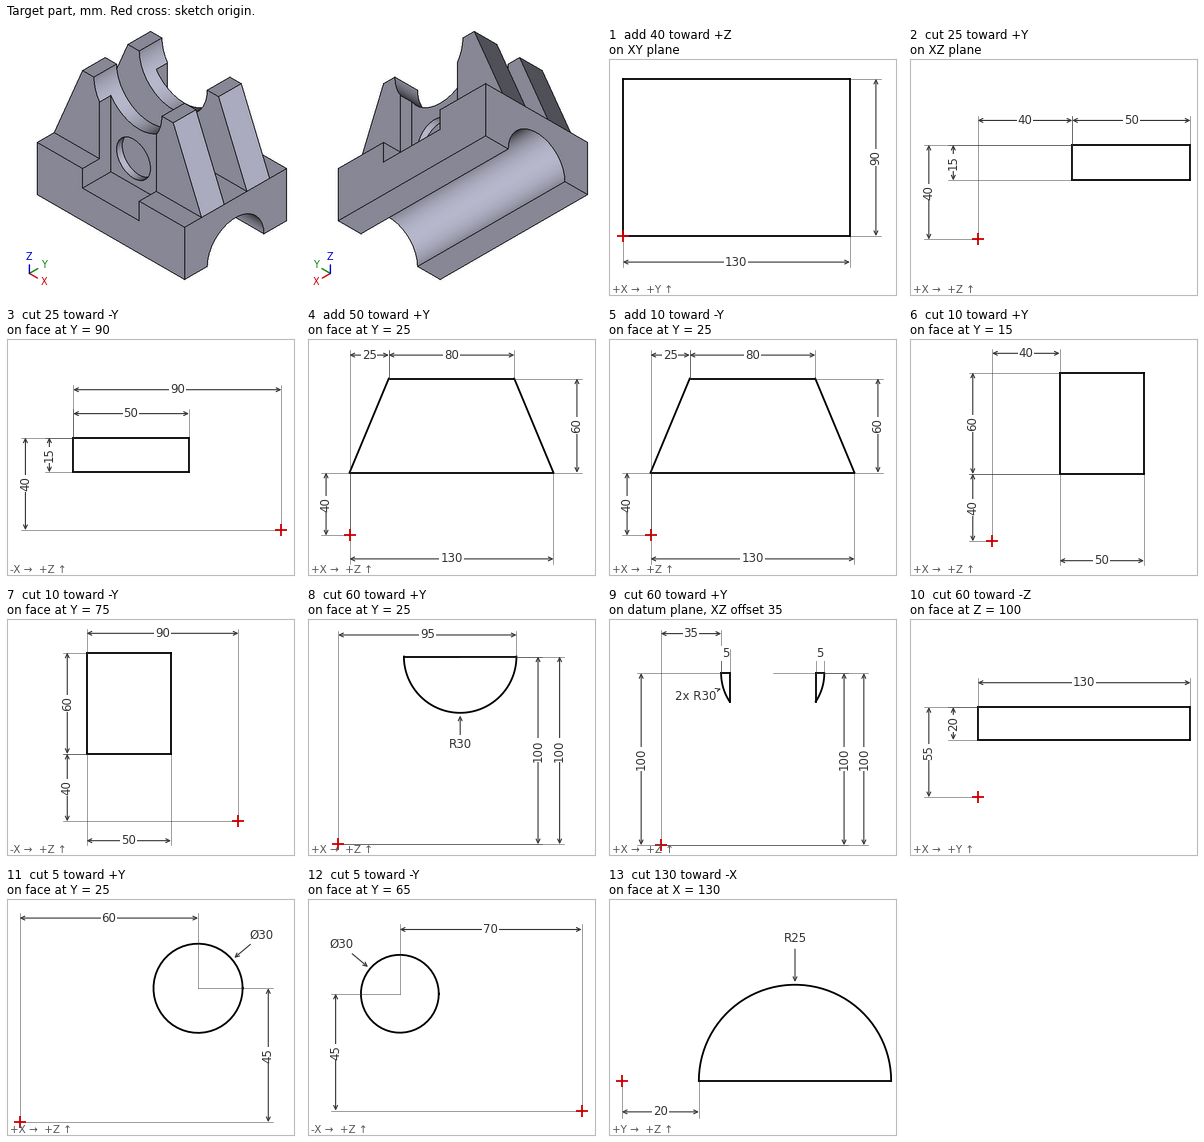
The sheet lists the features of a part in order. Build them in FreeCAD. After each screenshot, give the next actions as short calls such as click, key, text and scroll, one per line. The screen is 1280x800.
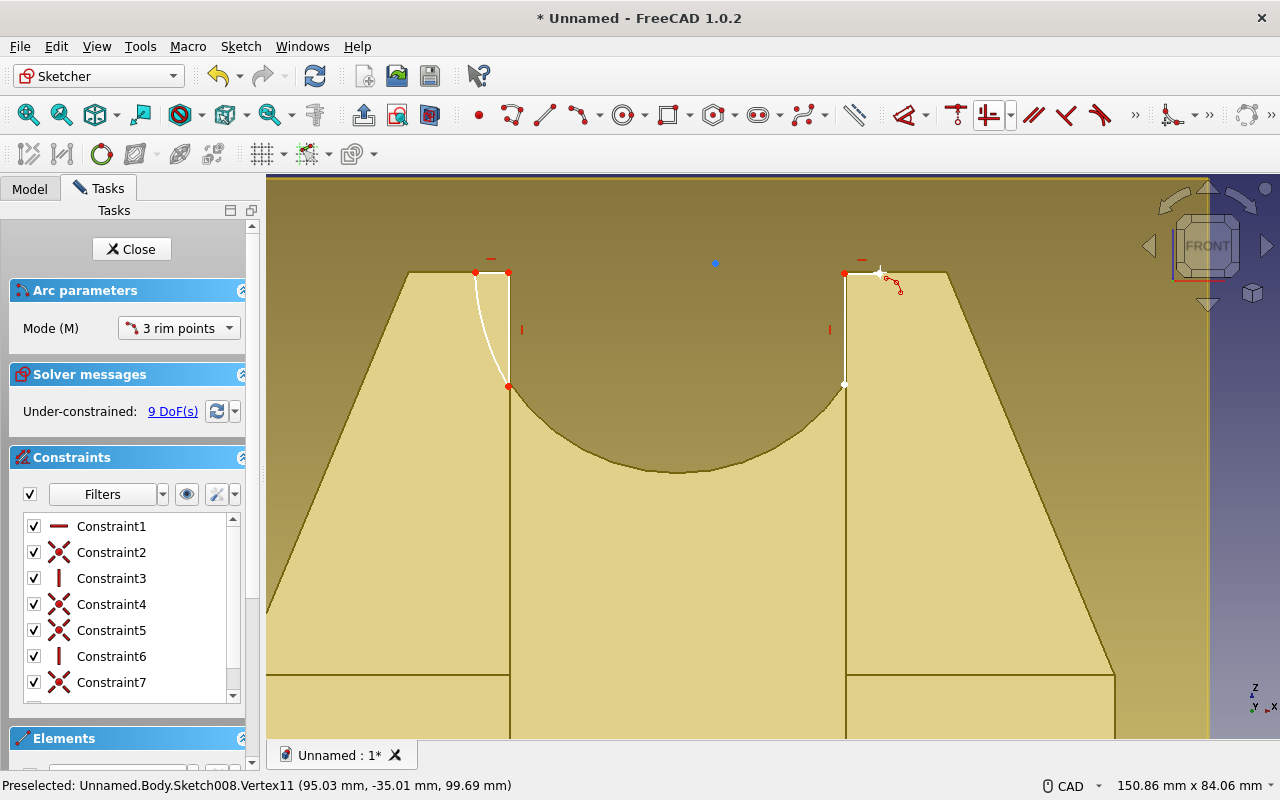
click(880, 274)
click(845, 385)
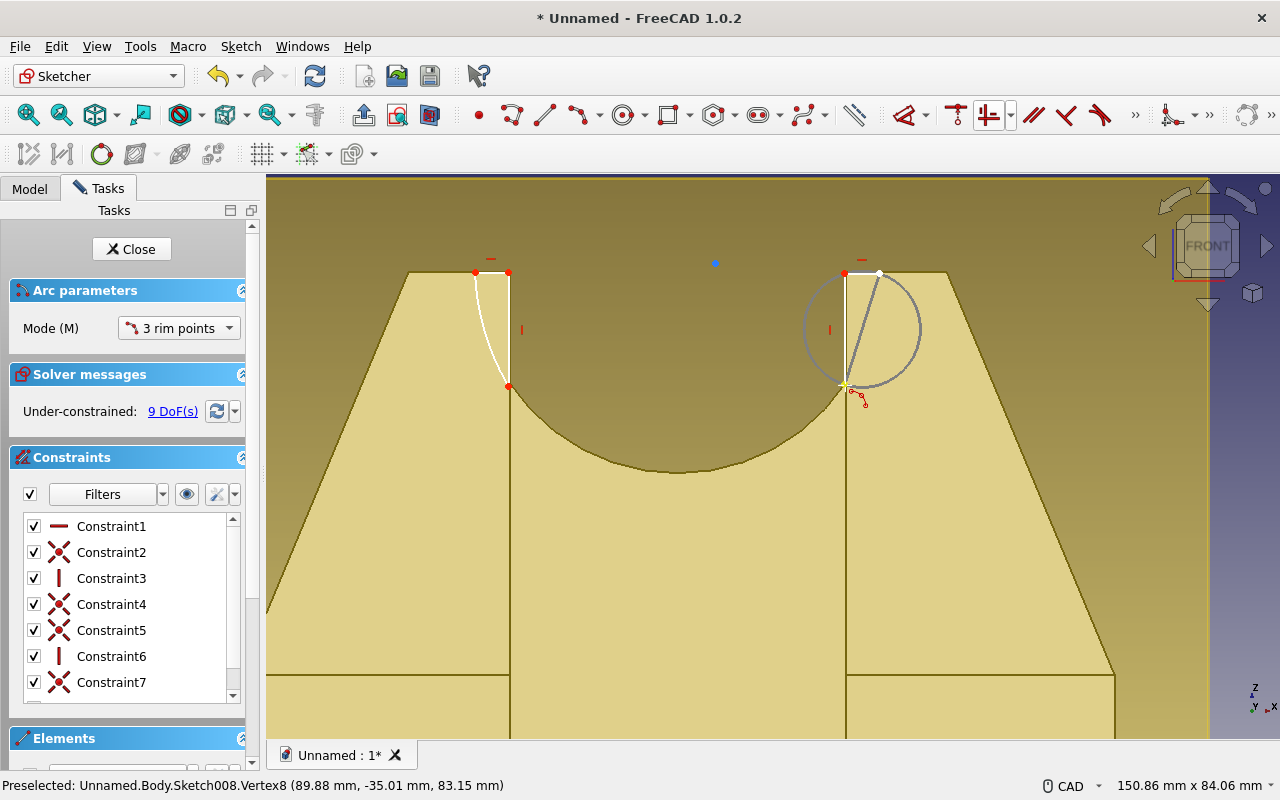
scroll(871, 330, up, 4)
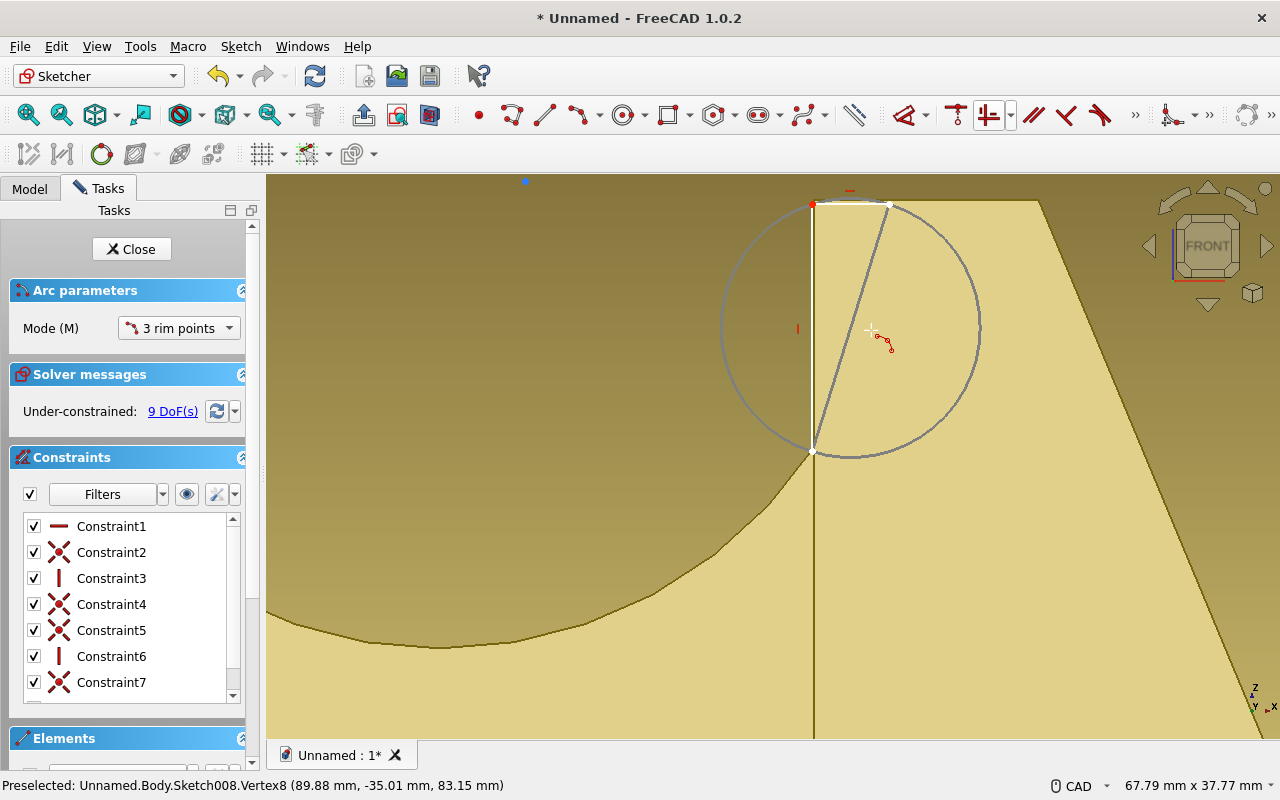
click(870, 329)
key(Escape)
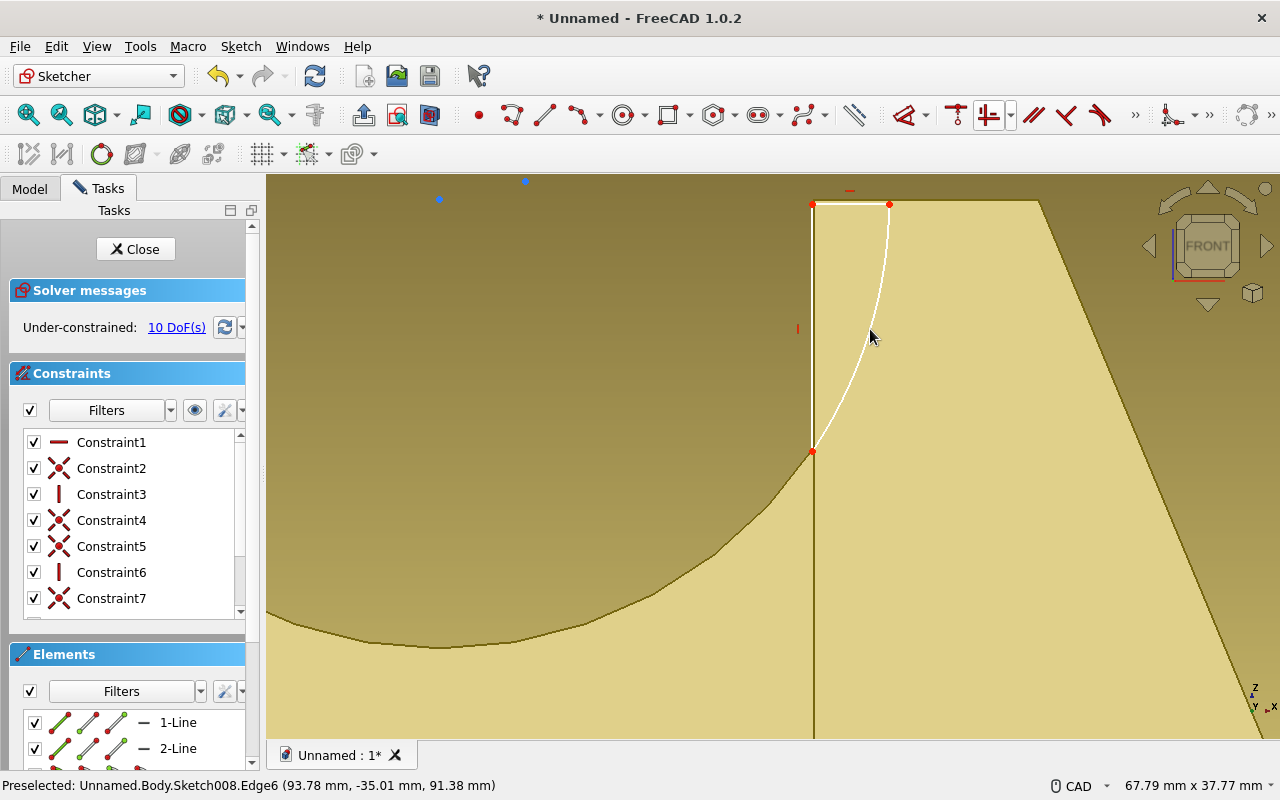
scroll(877, 296, down, 7)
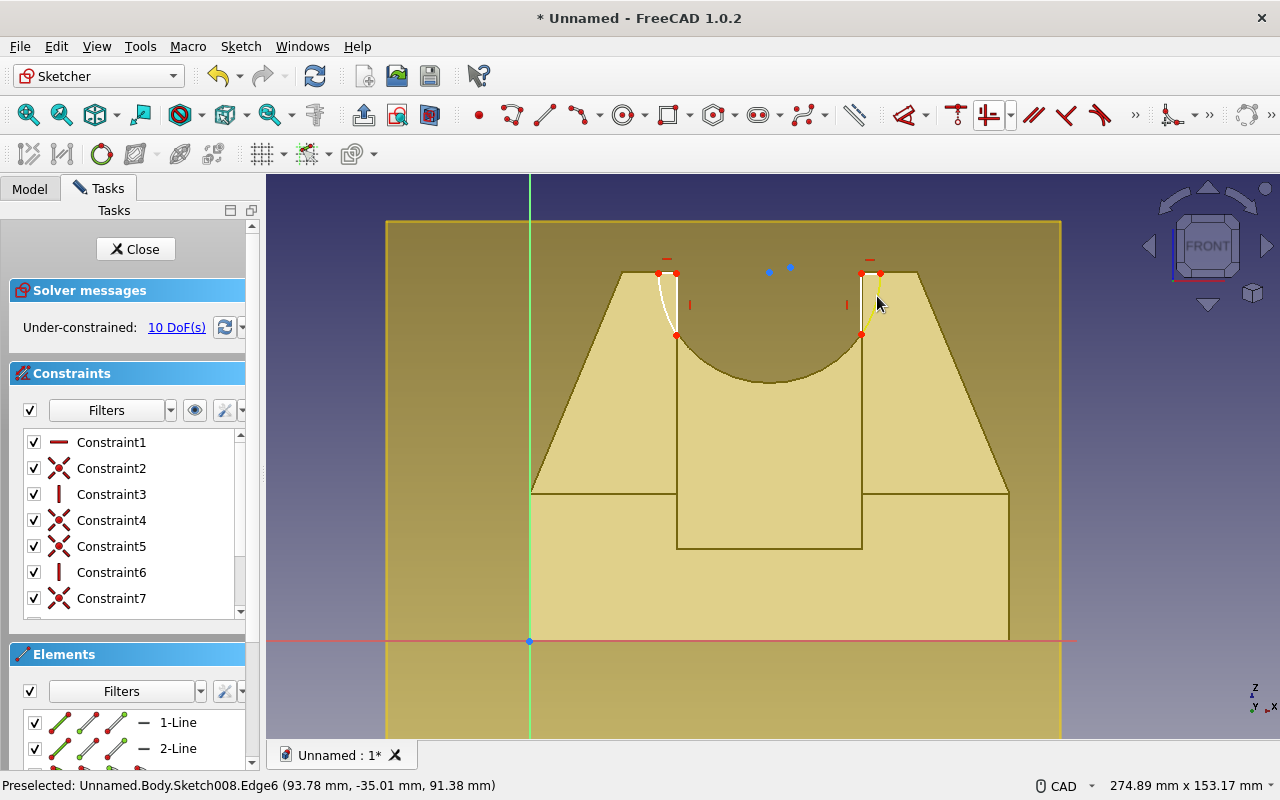
click(661, 293)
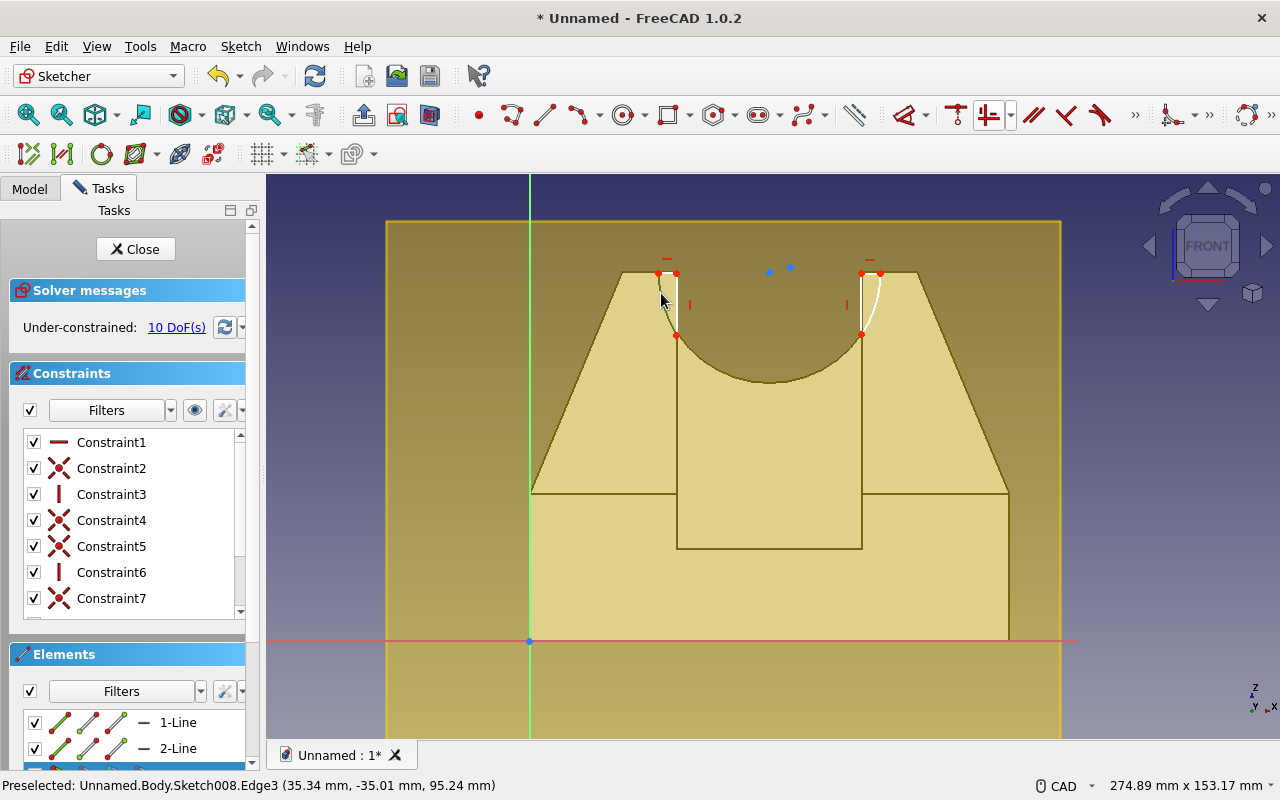
scroll(871, 318, up, 2)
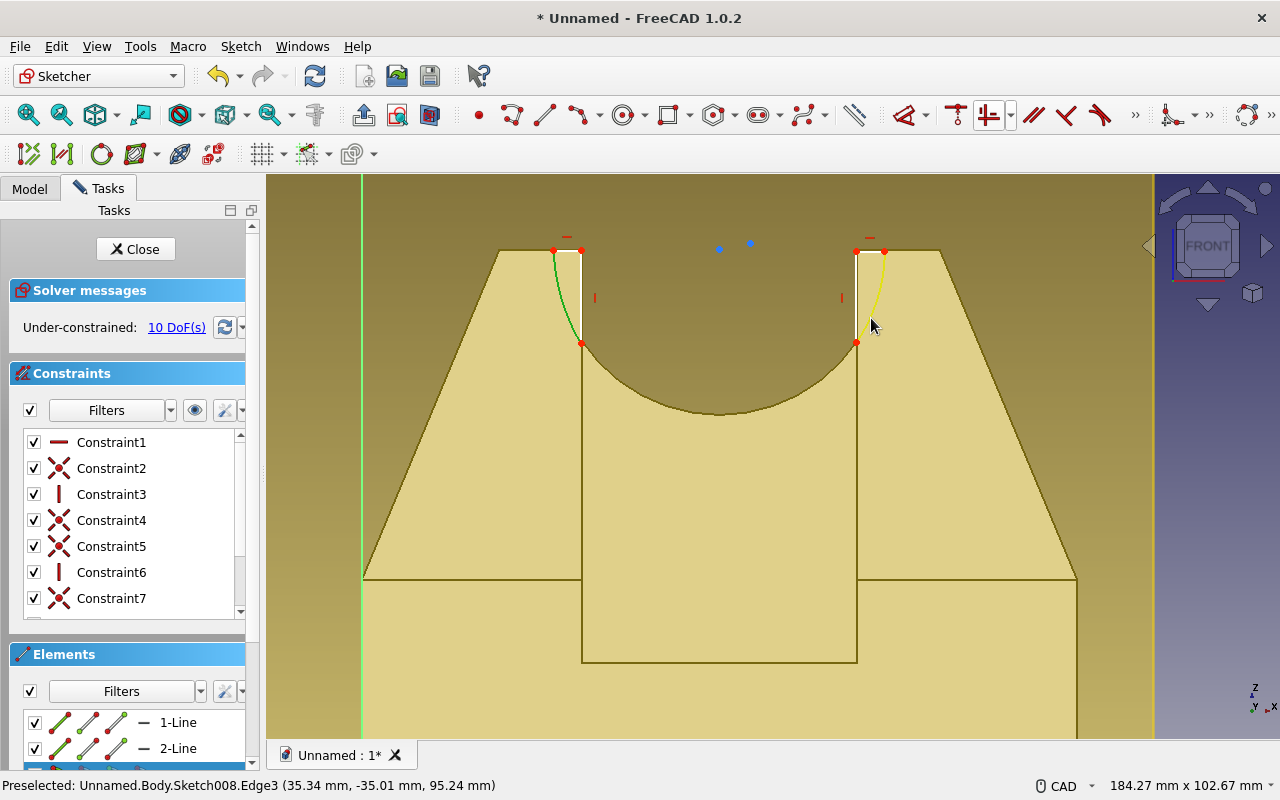
click(871, 317)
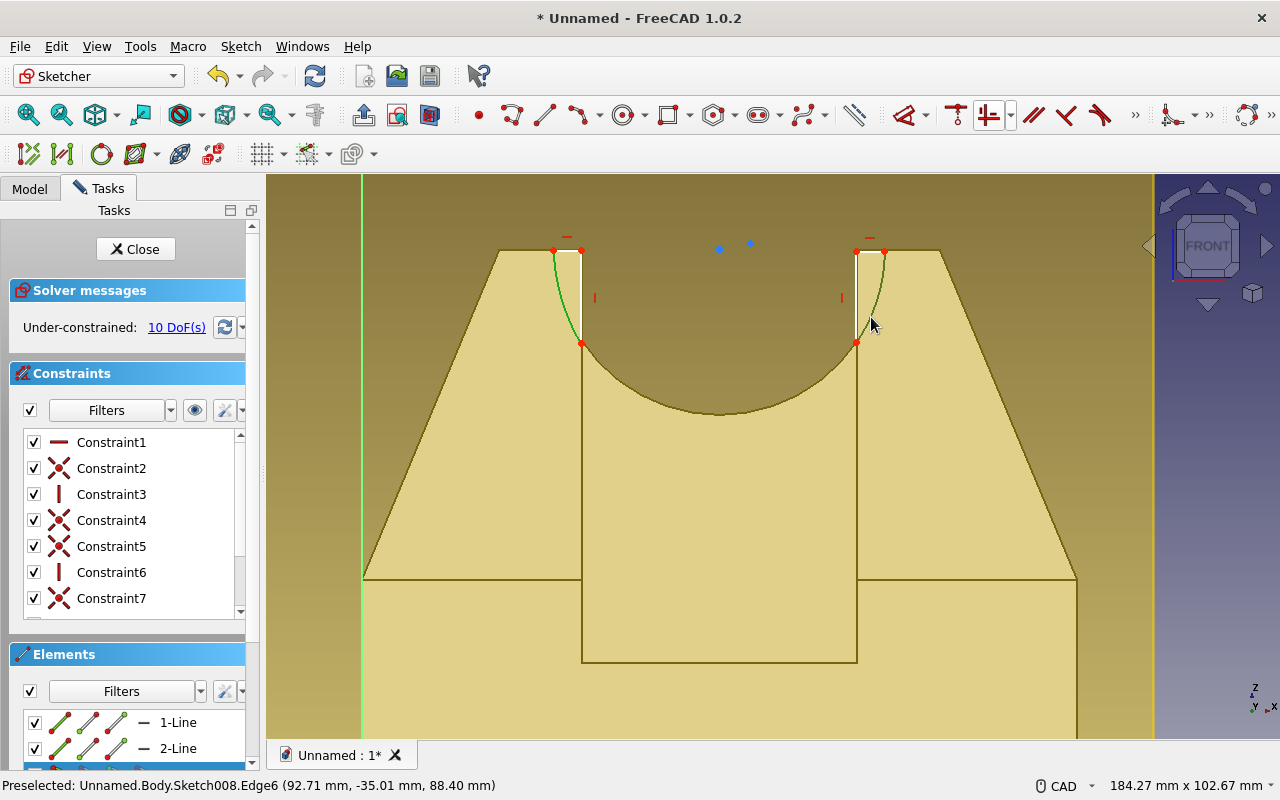
key(c)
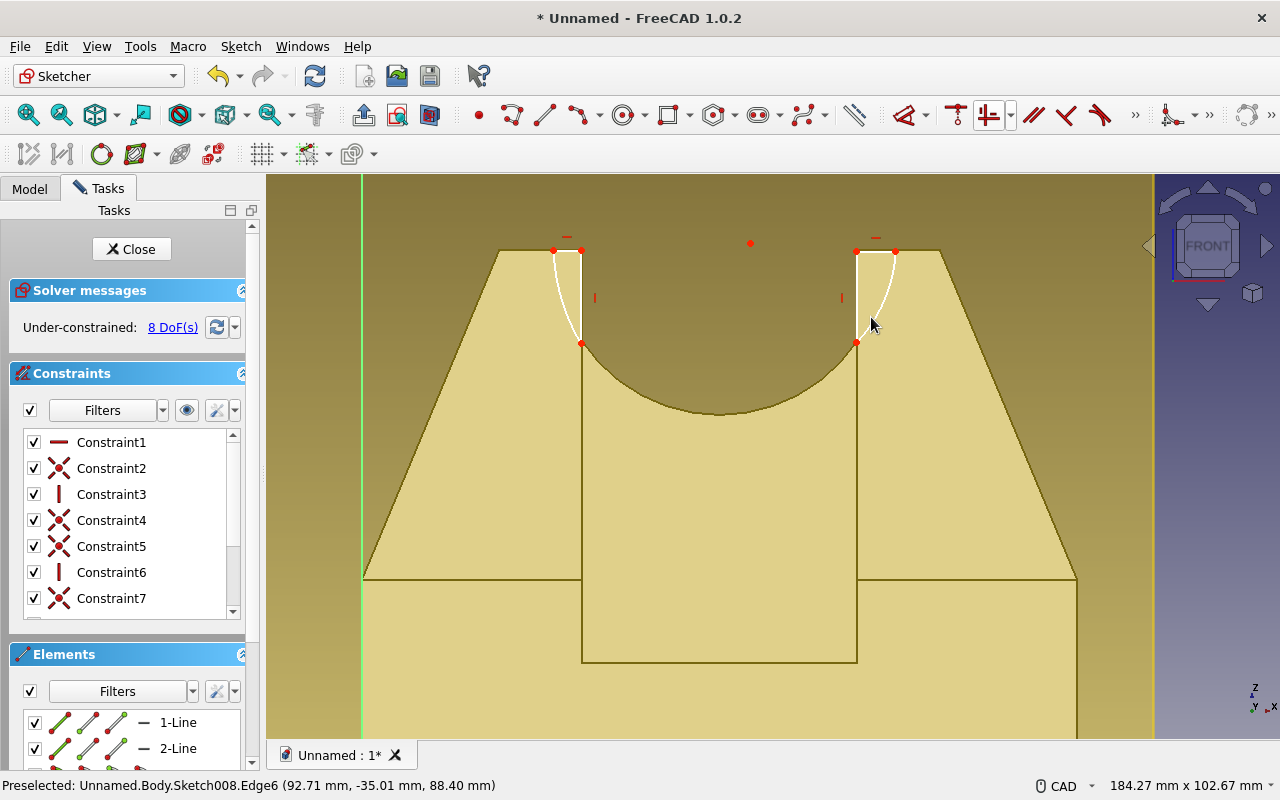
click(557, 280)